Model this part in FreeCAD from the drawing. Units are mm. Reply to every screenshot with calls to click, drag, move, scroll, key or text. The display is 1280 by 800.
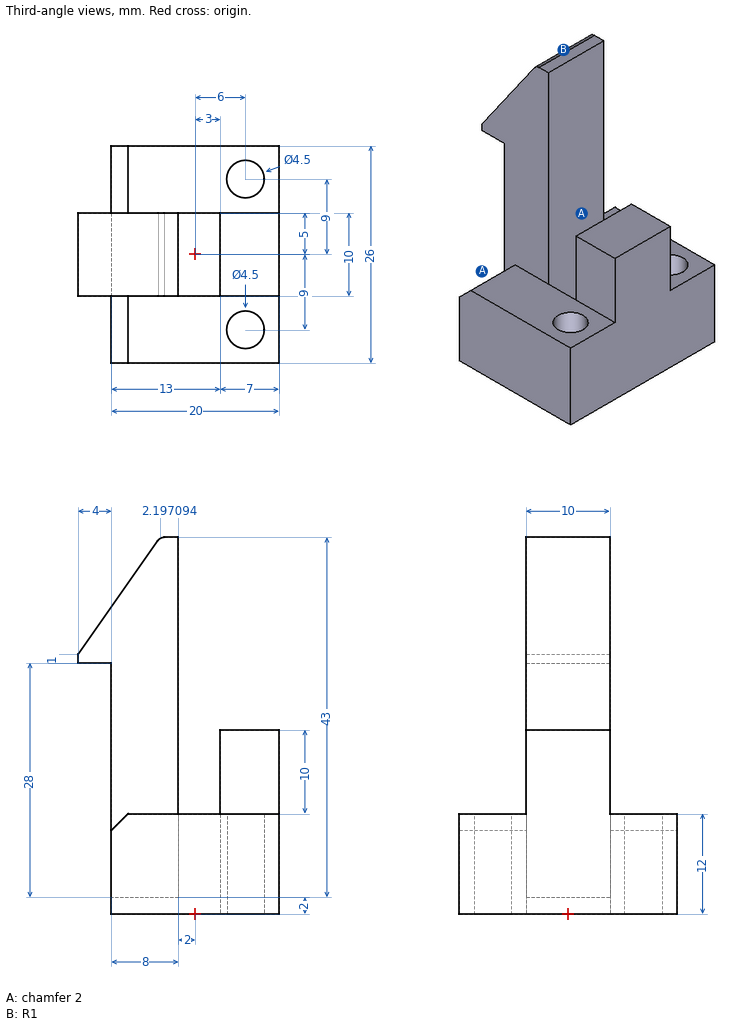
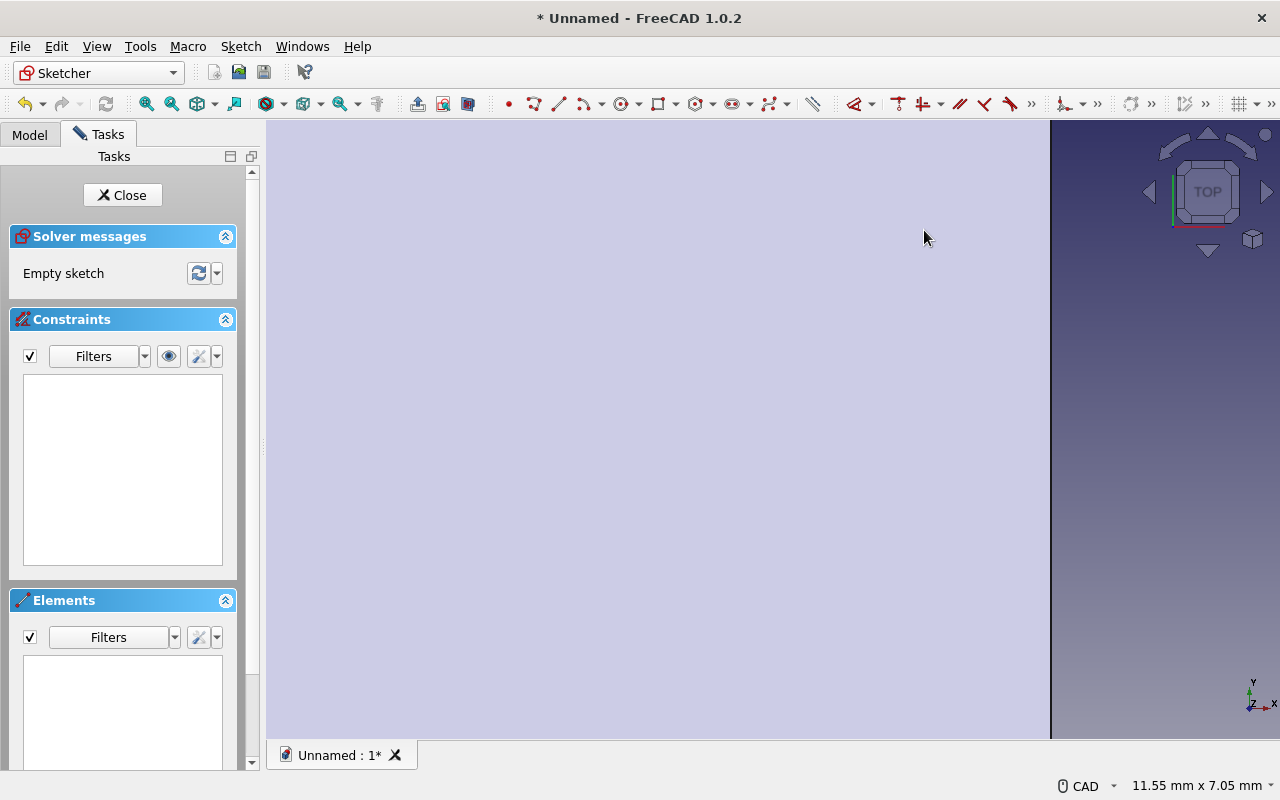
key(g)
key(c)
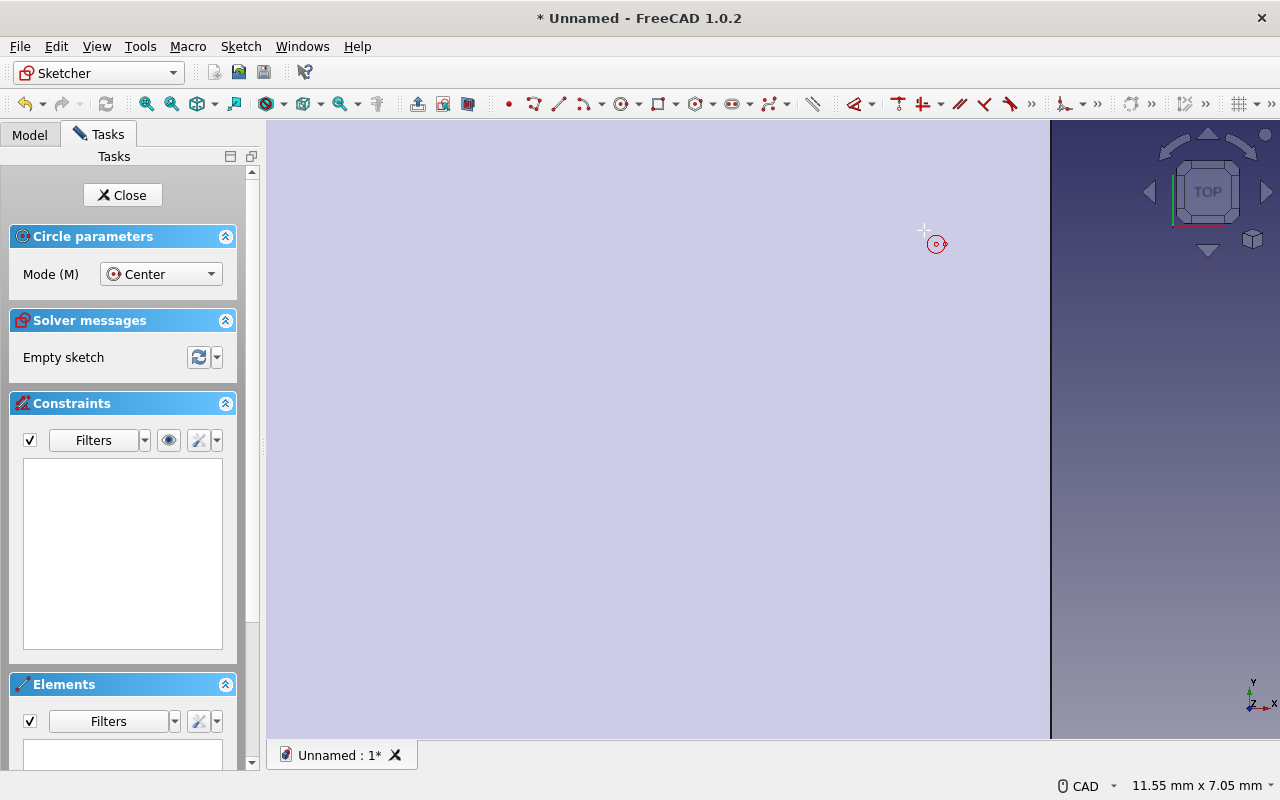
click(700, 427)
click(840, 288)
key(Escape)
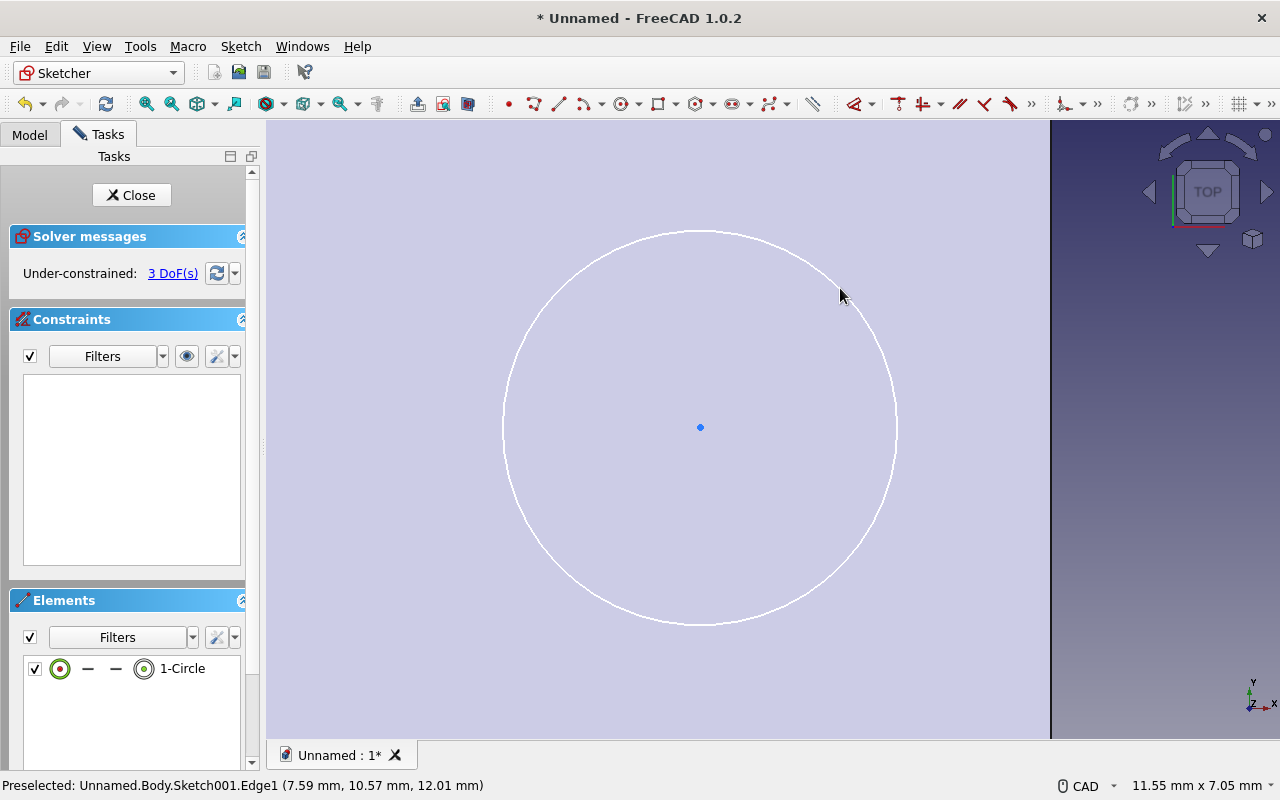
key(d)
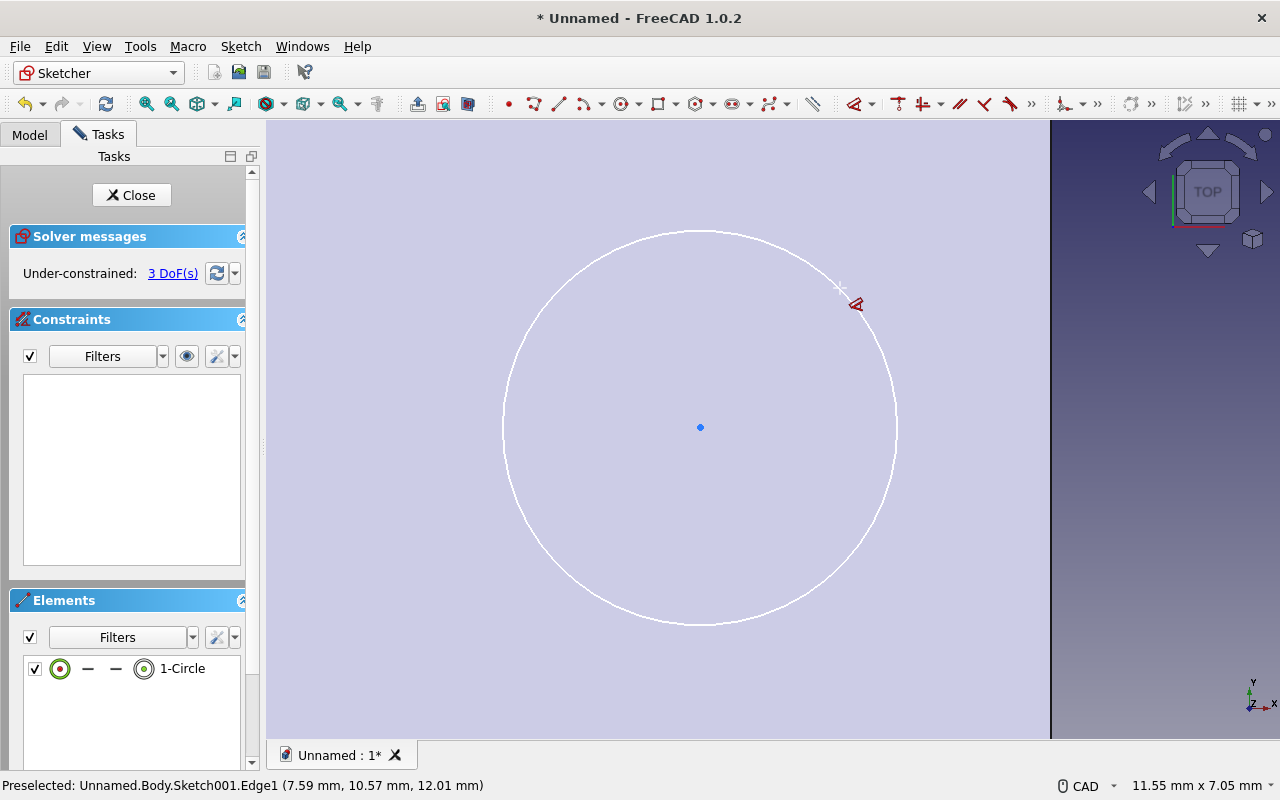
click(839, 288)
click(862, 265)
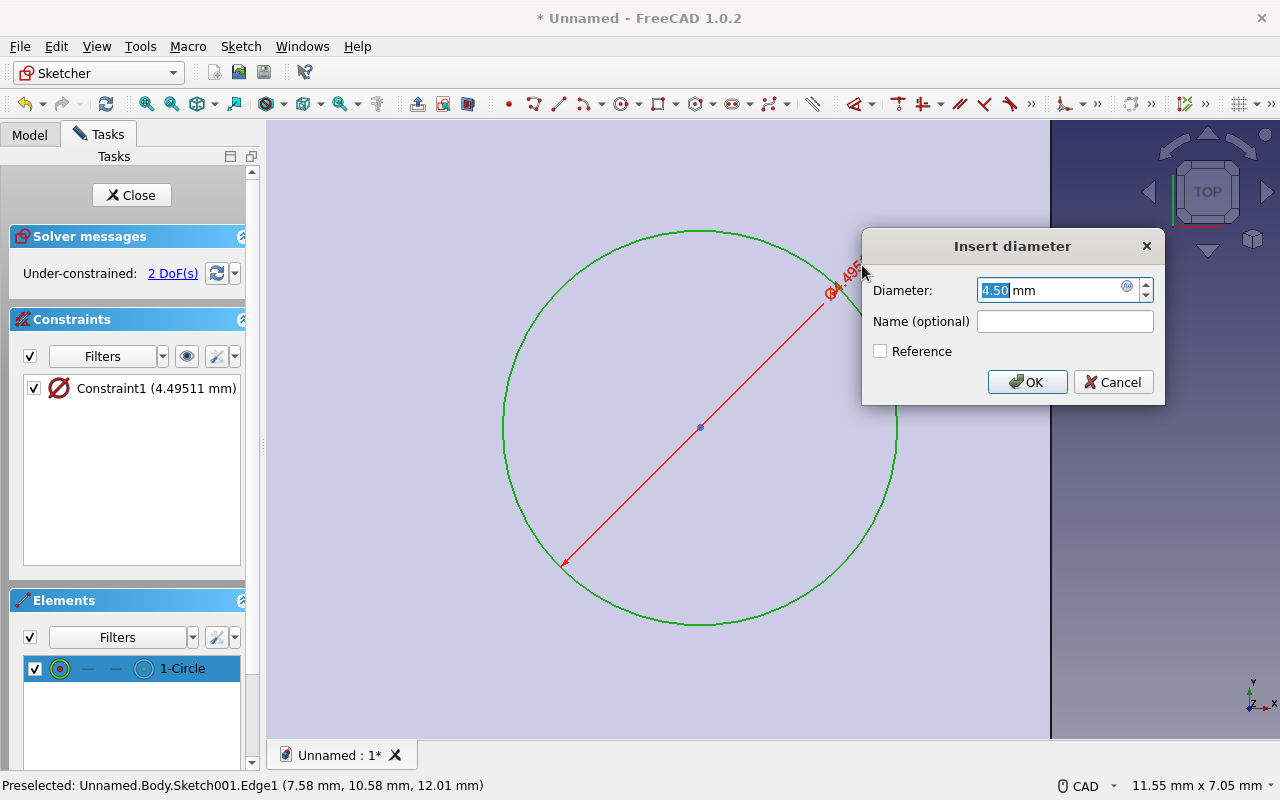
text(4.5)
key(Return)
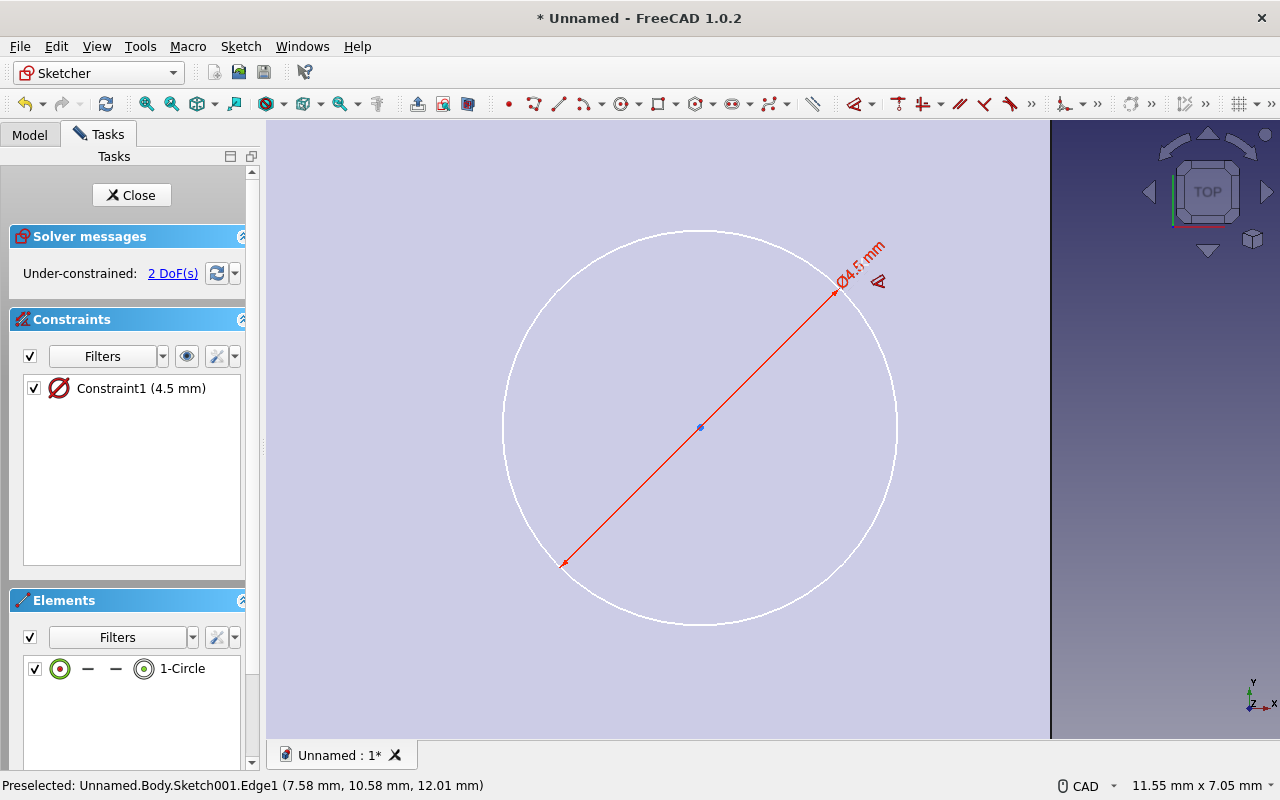
click(700, 428)
click(404, 394)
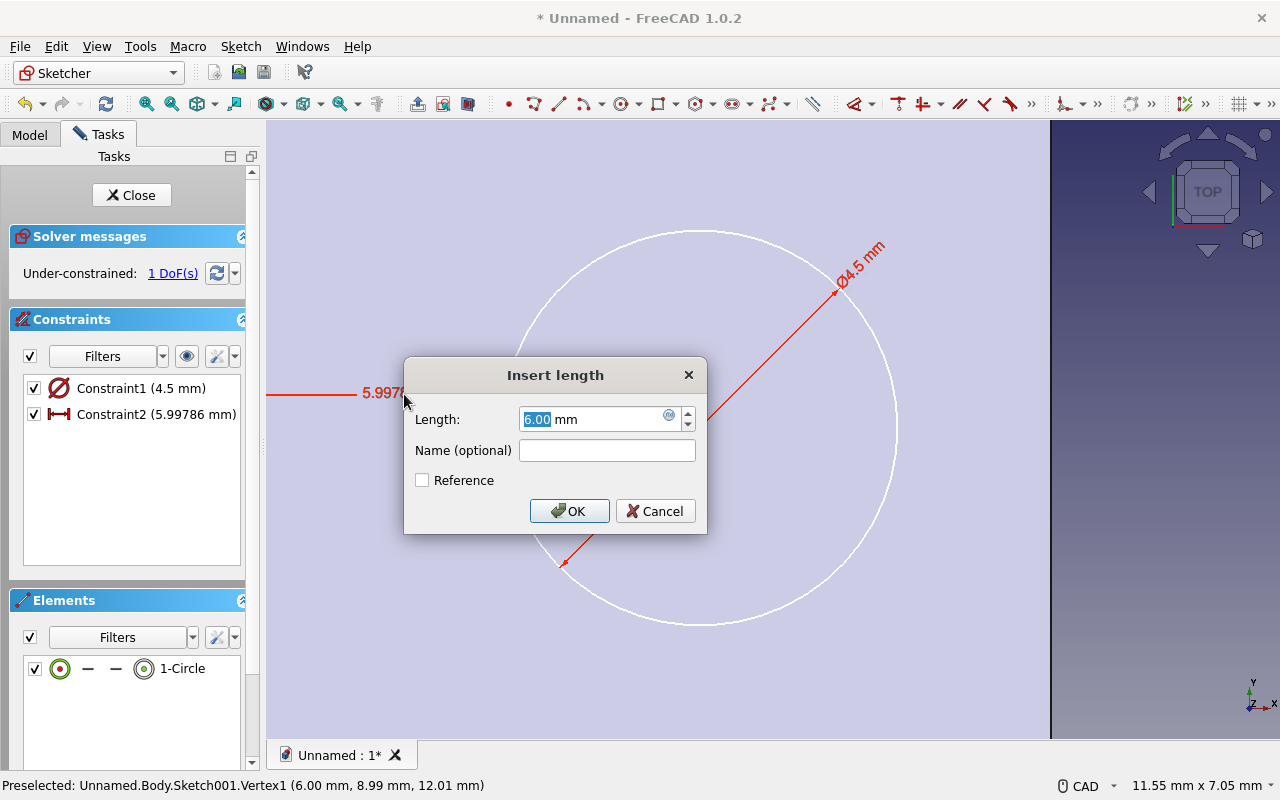
text(6)
key(Return)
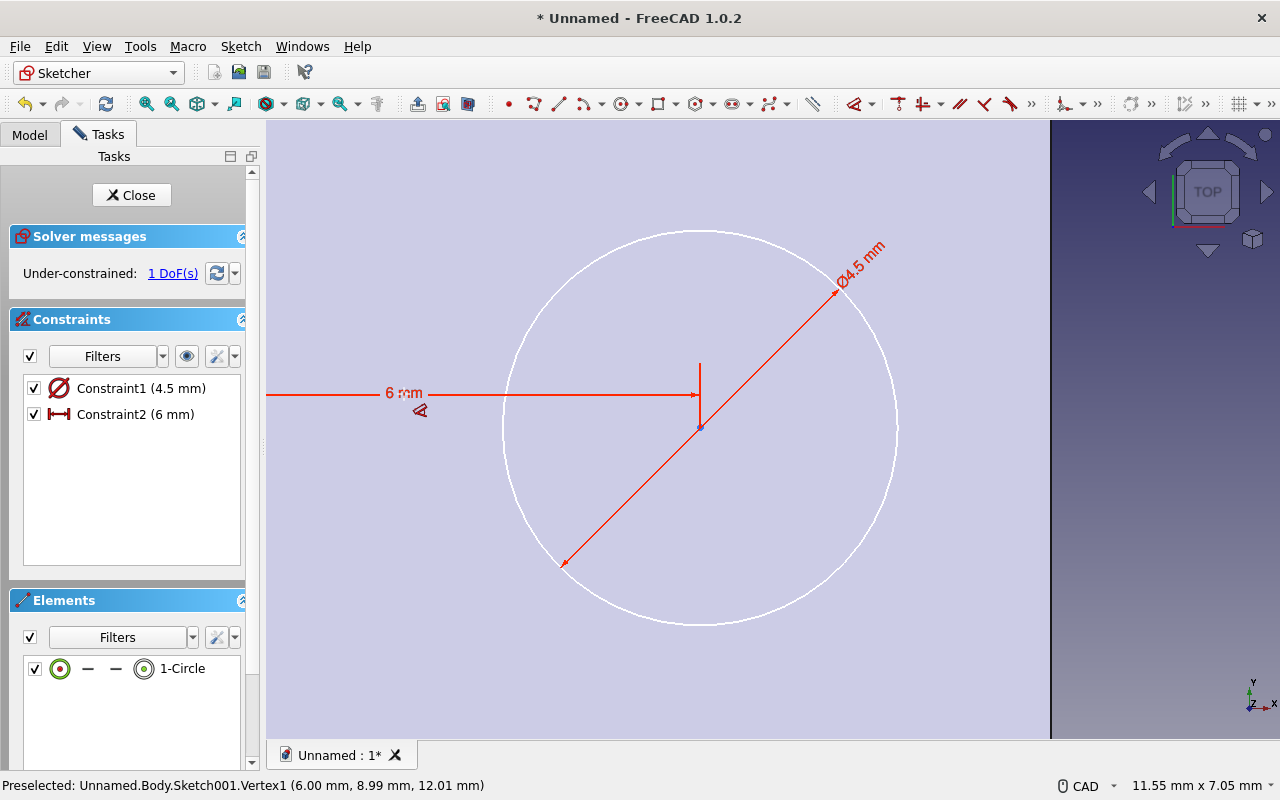
click(700, 428)
click(734, 569)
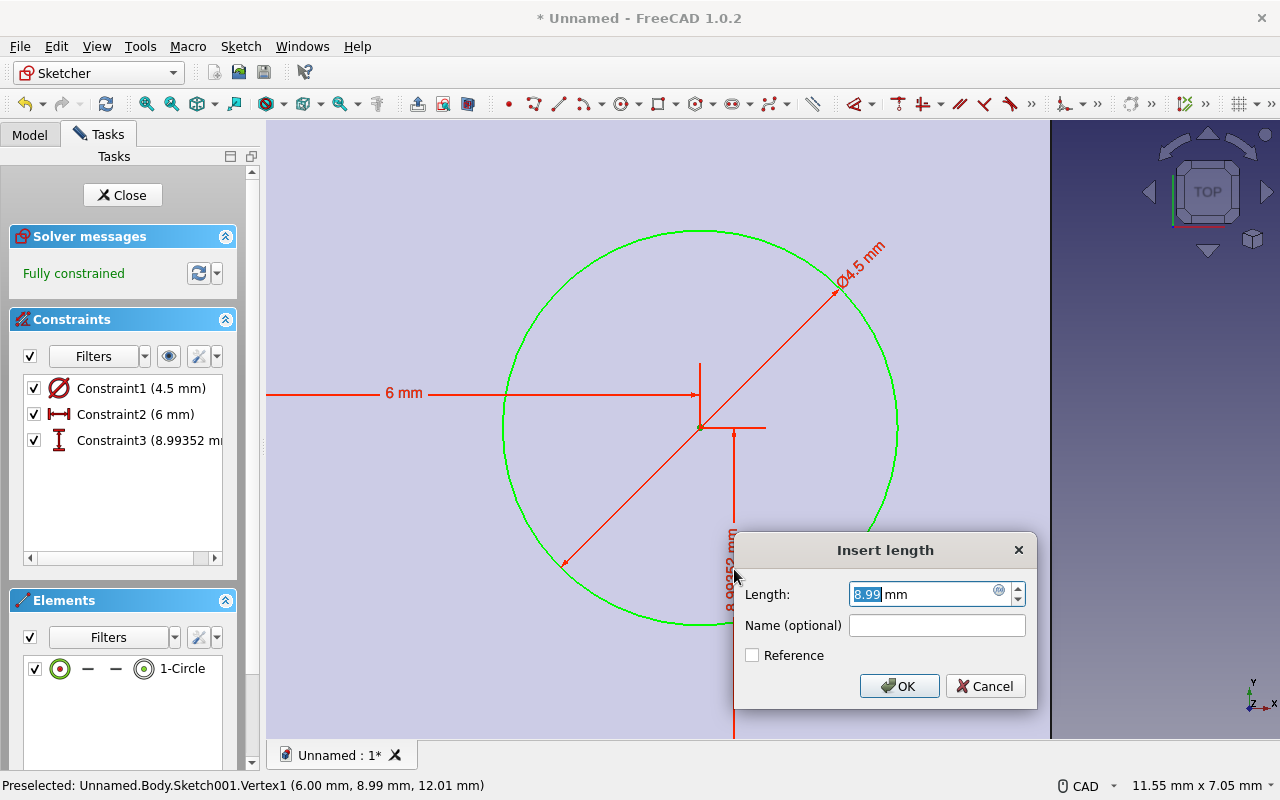
text(9)
key(Return)
key(Escape)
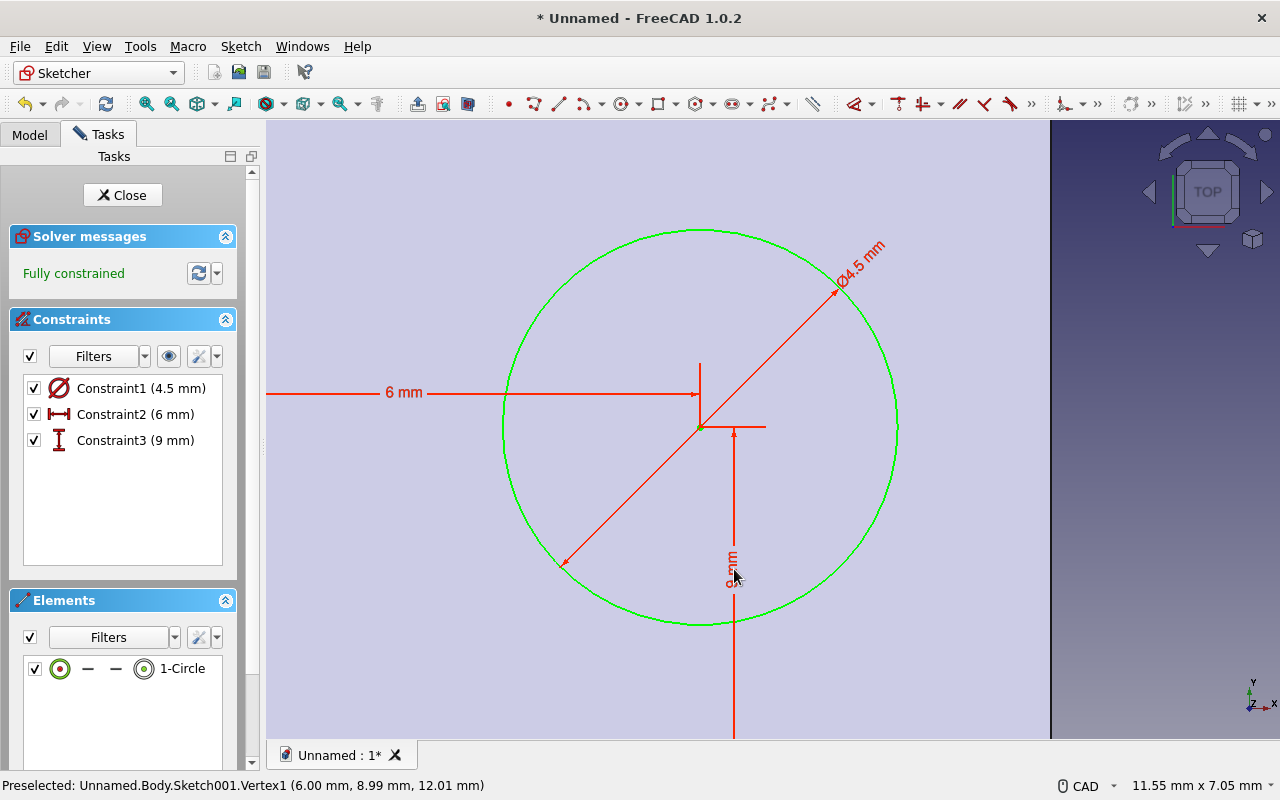
click(123, 195)